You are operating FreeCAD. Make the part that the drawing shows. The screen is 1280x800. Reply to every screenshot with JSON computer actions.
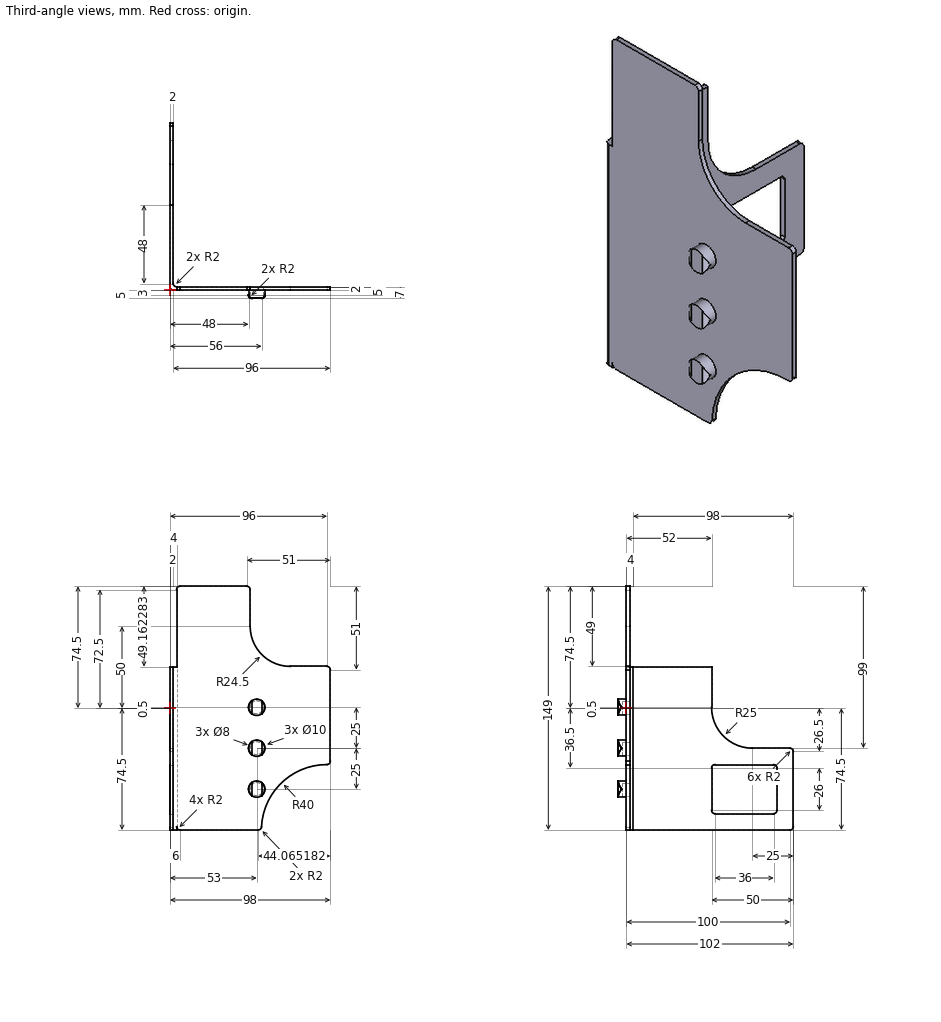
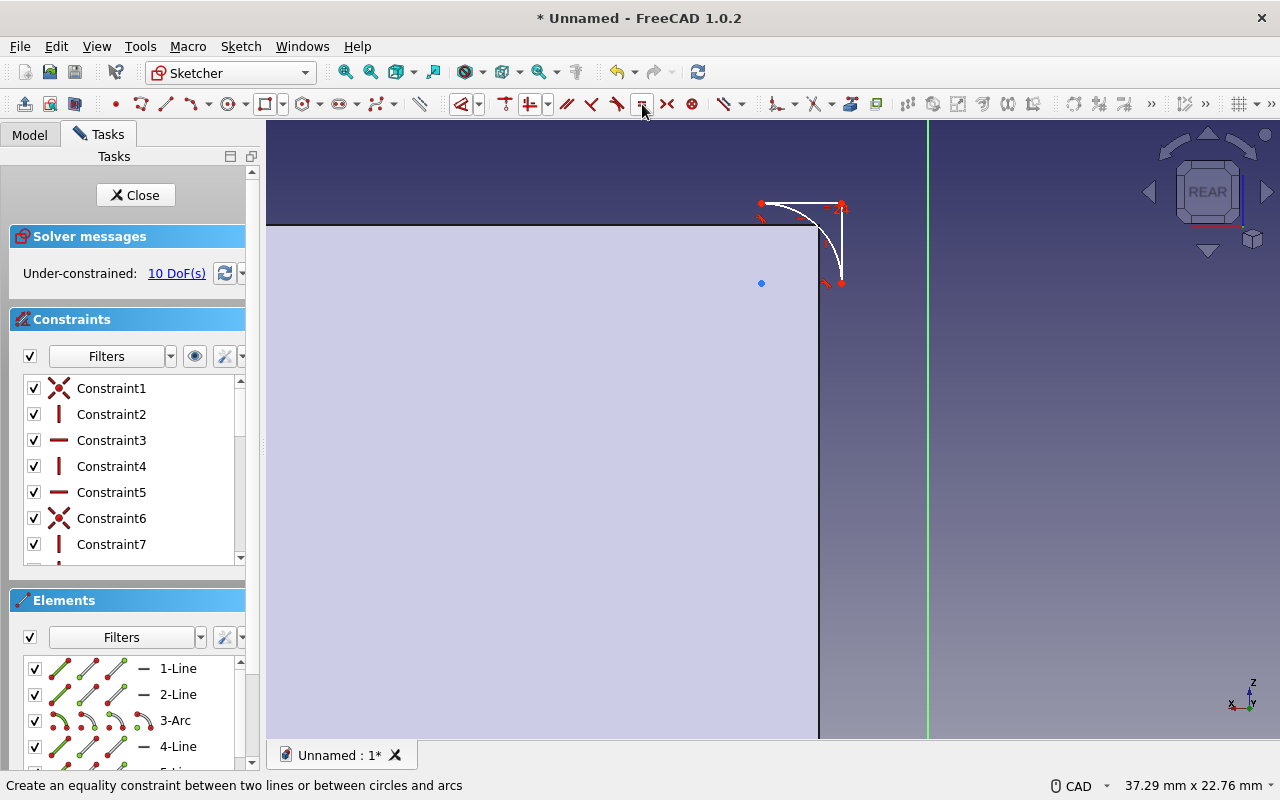
{"action": "scroll", "coordinate": [815, 248], "scroll_direction": "down", "scroll_amount": 12}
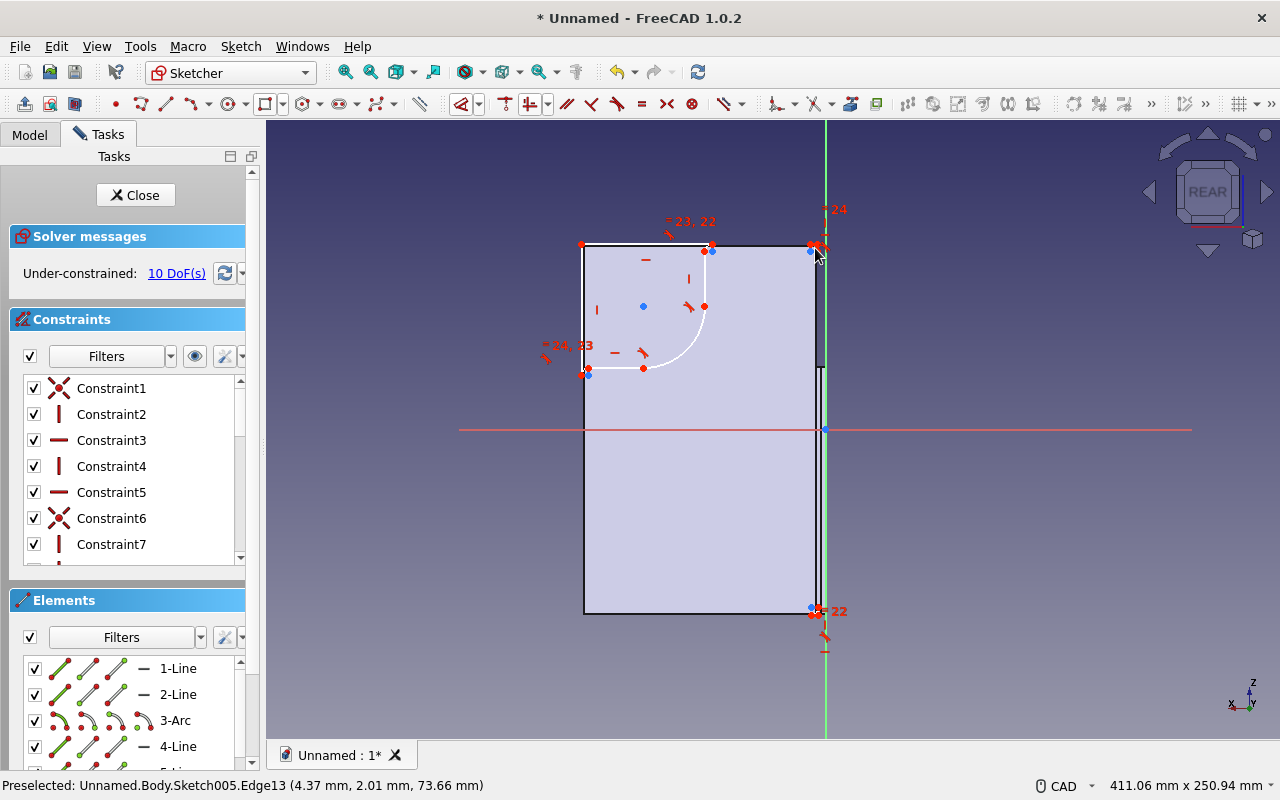
{"action": "scroll", "coordinate": [816, 613], "scroll_direction": "up", "scroll_amount": 11}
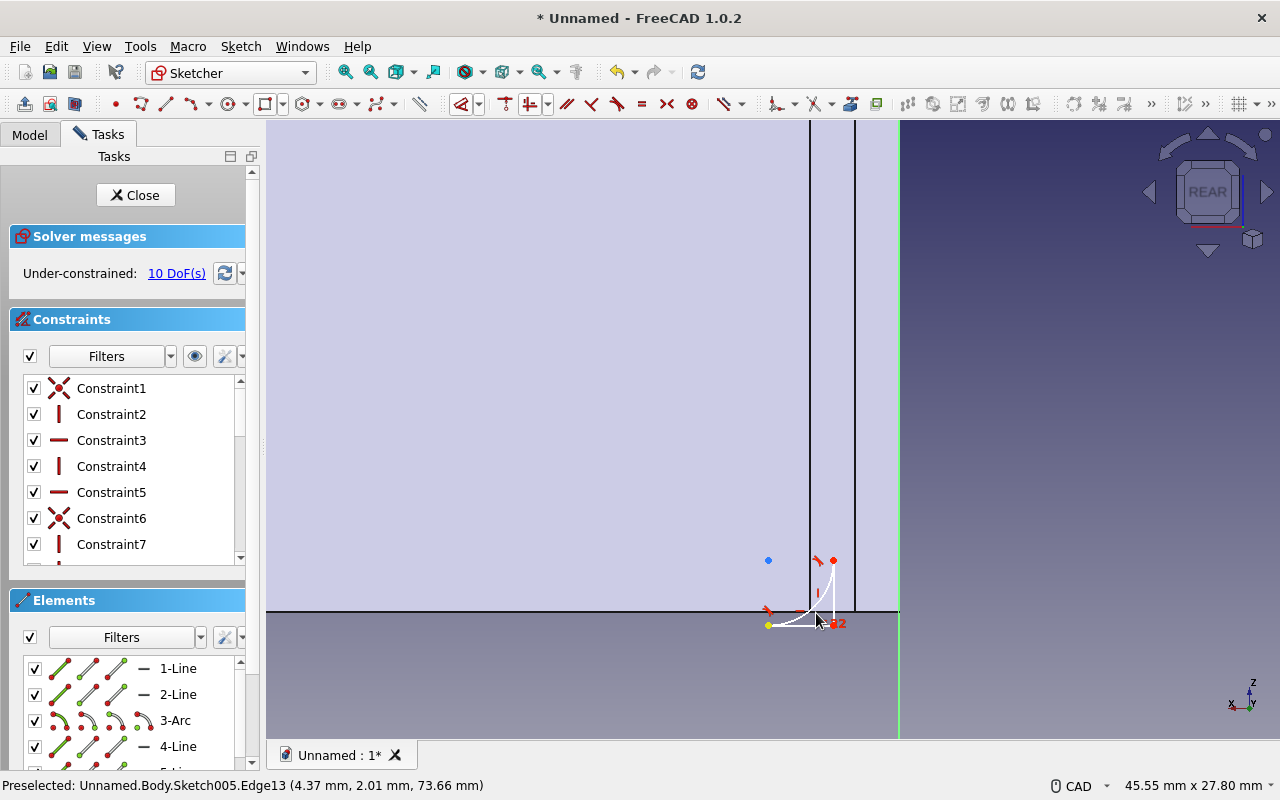
{"action": "left_click", "coordinate": [815, 606]}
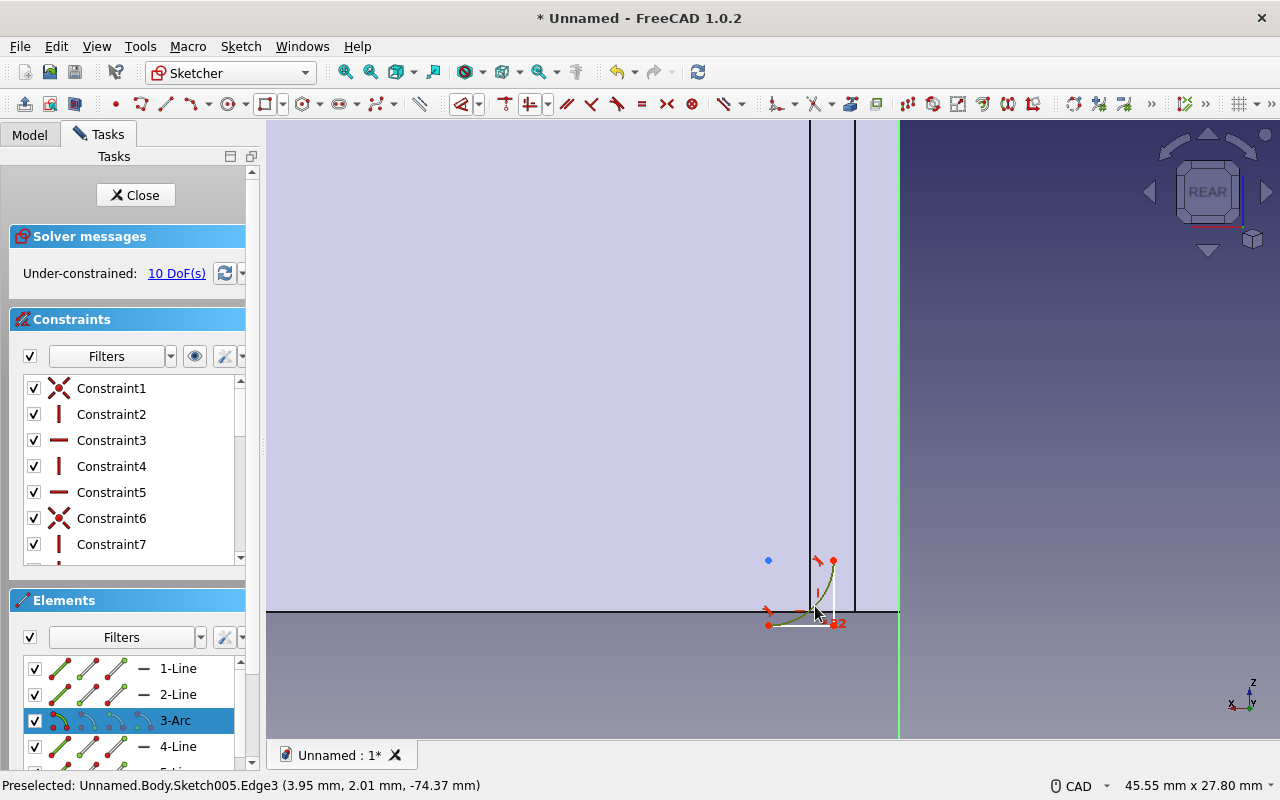
{"action": "key", "text": "k r"}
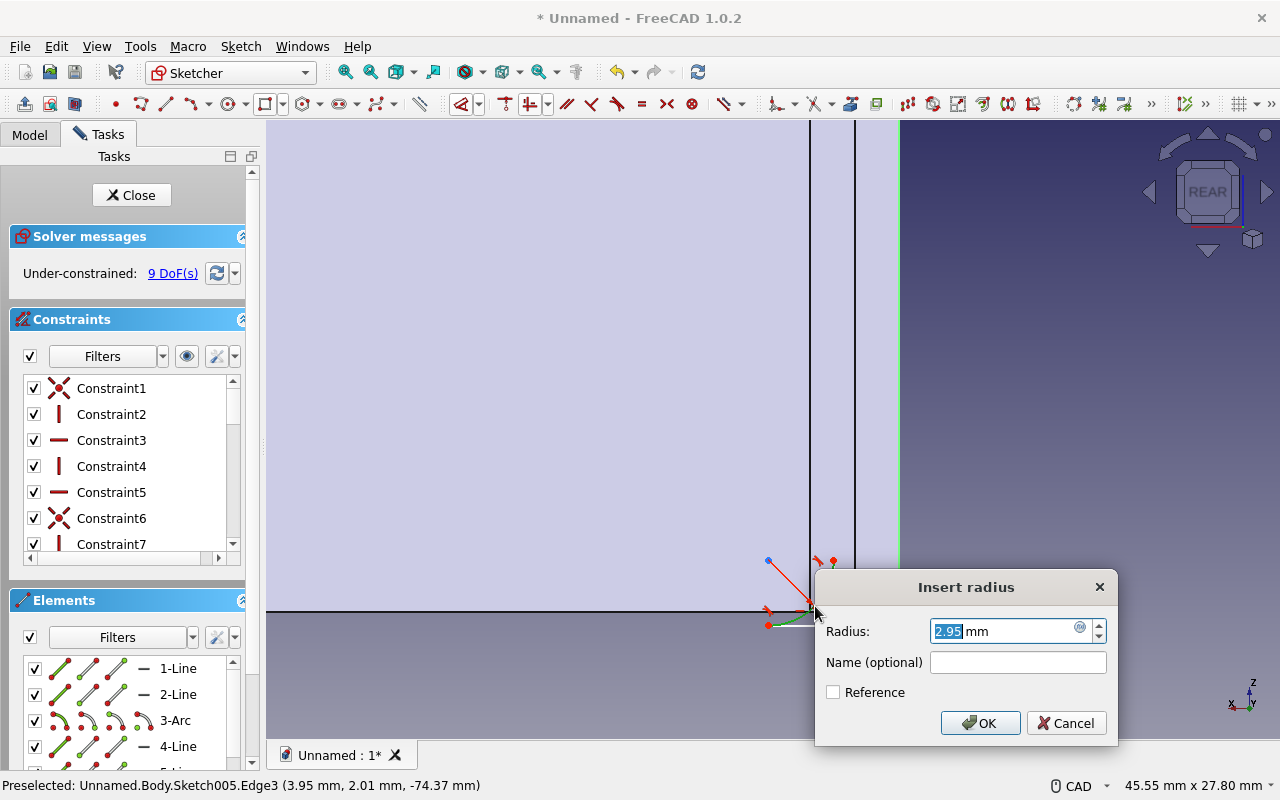
{"action": "type", "text": "2"}
{"action": "key", "text": "Return"}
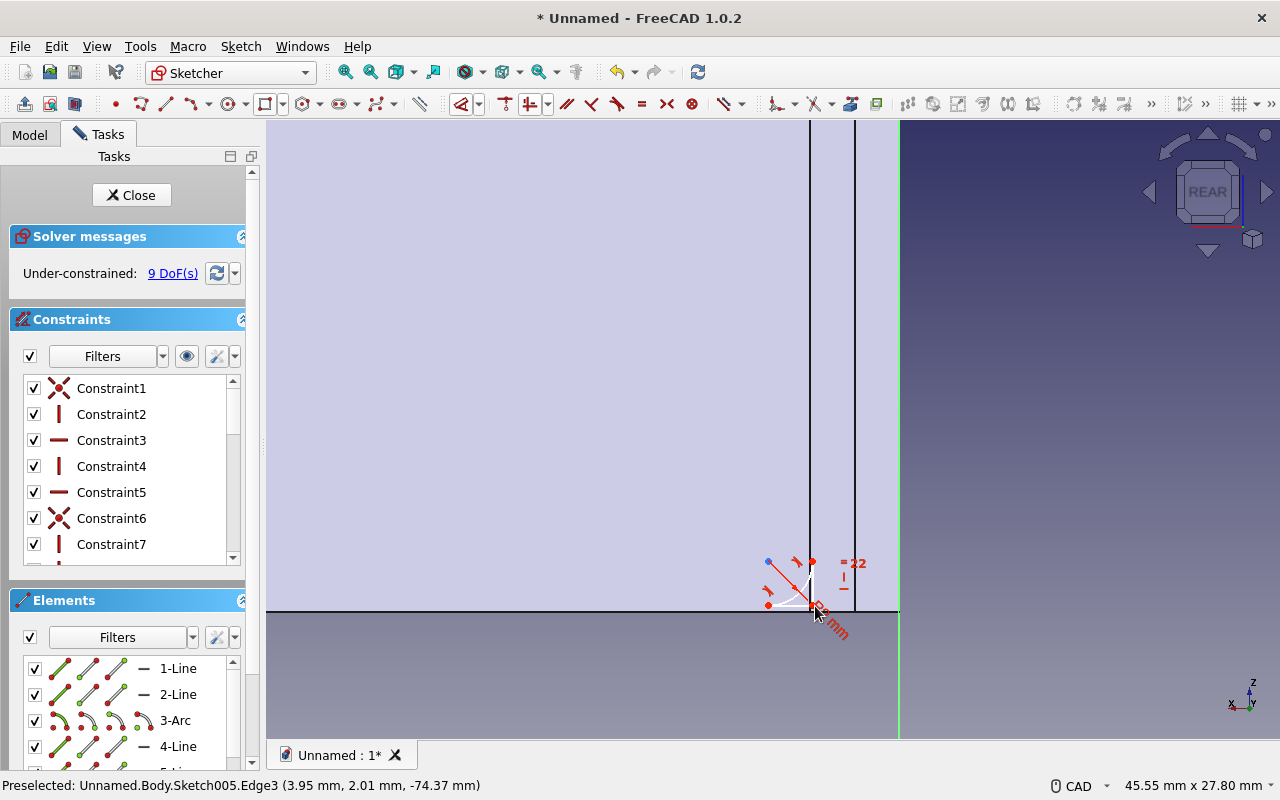
{"action": "scroll", "coordinate": [816, 613], "scroll_direction": "down", "scroll_amount": 11}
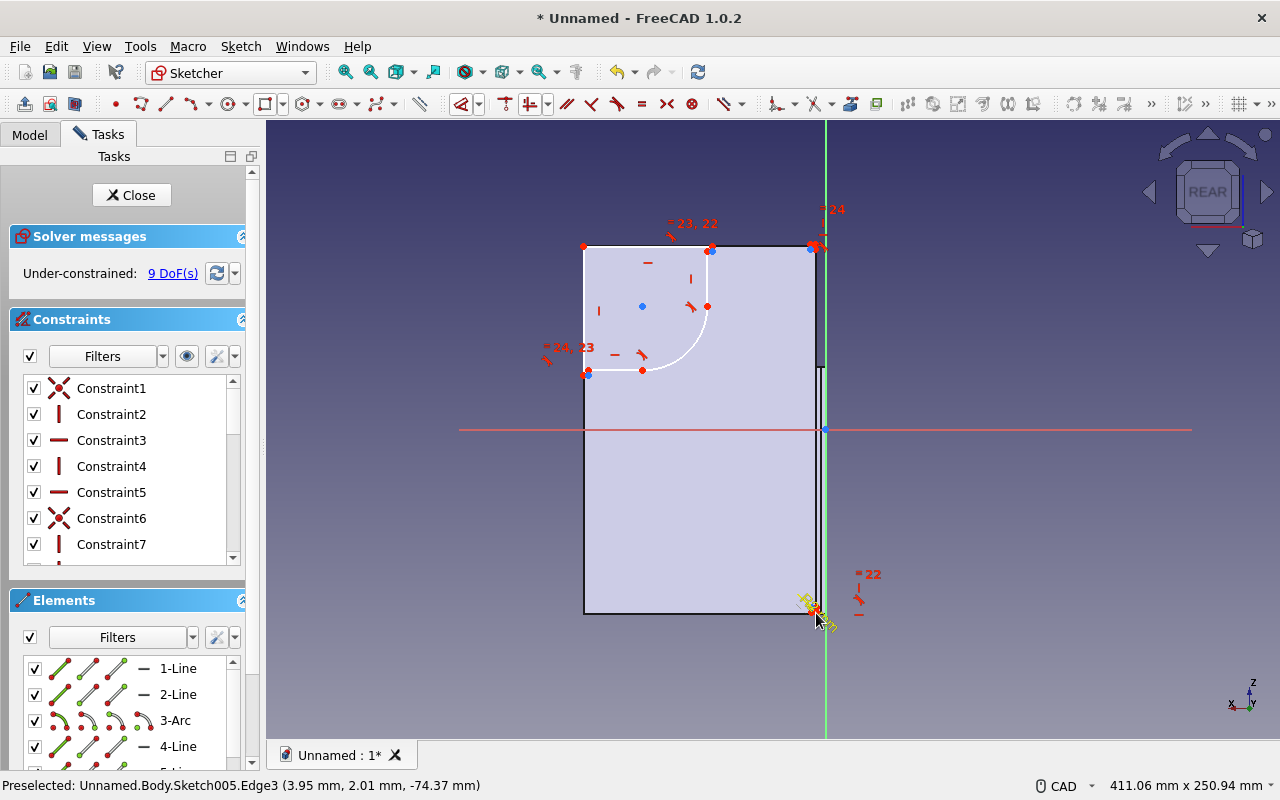
{"action": "left_click", "coordinate": [672, 363]}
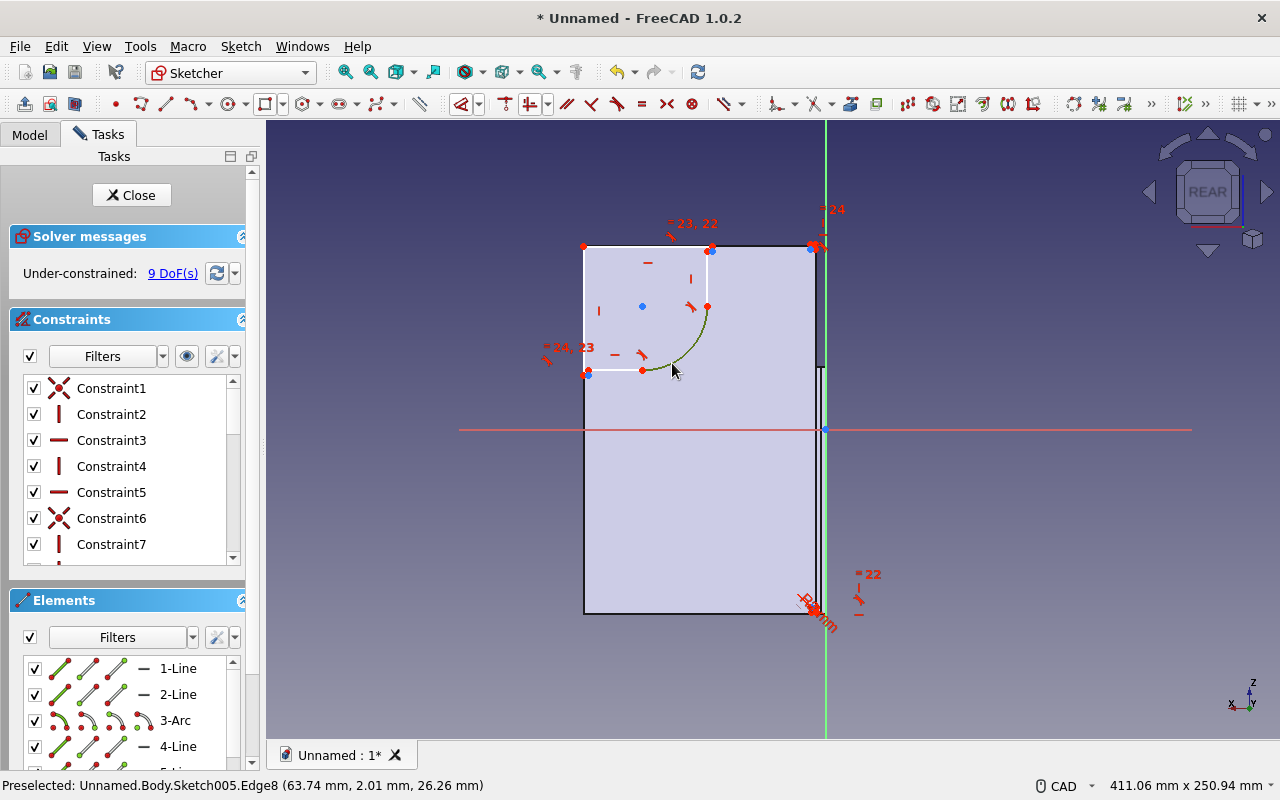
{"action": "key", "text": "k r"}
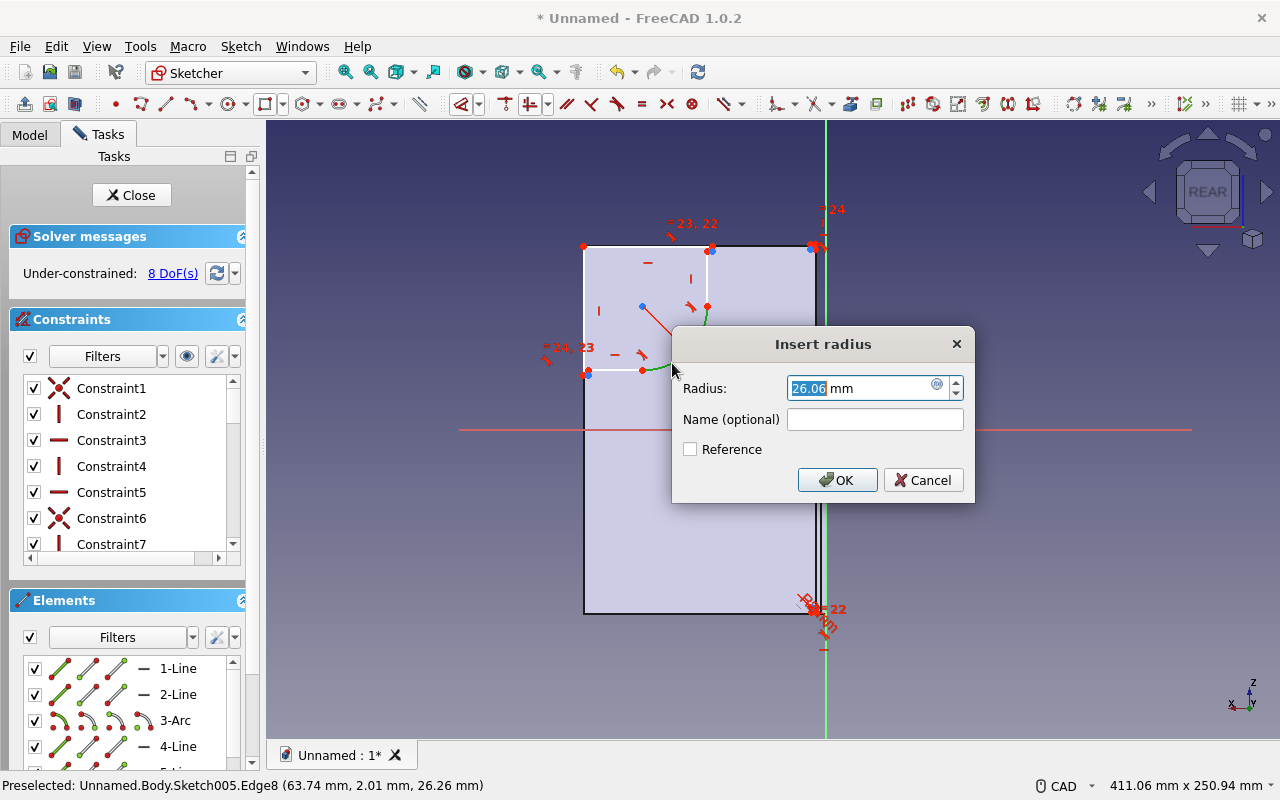
{"action": "type", "text": "24.5"}
{"action": "key", "text": "Return"}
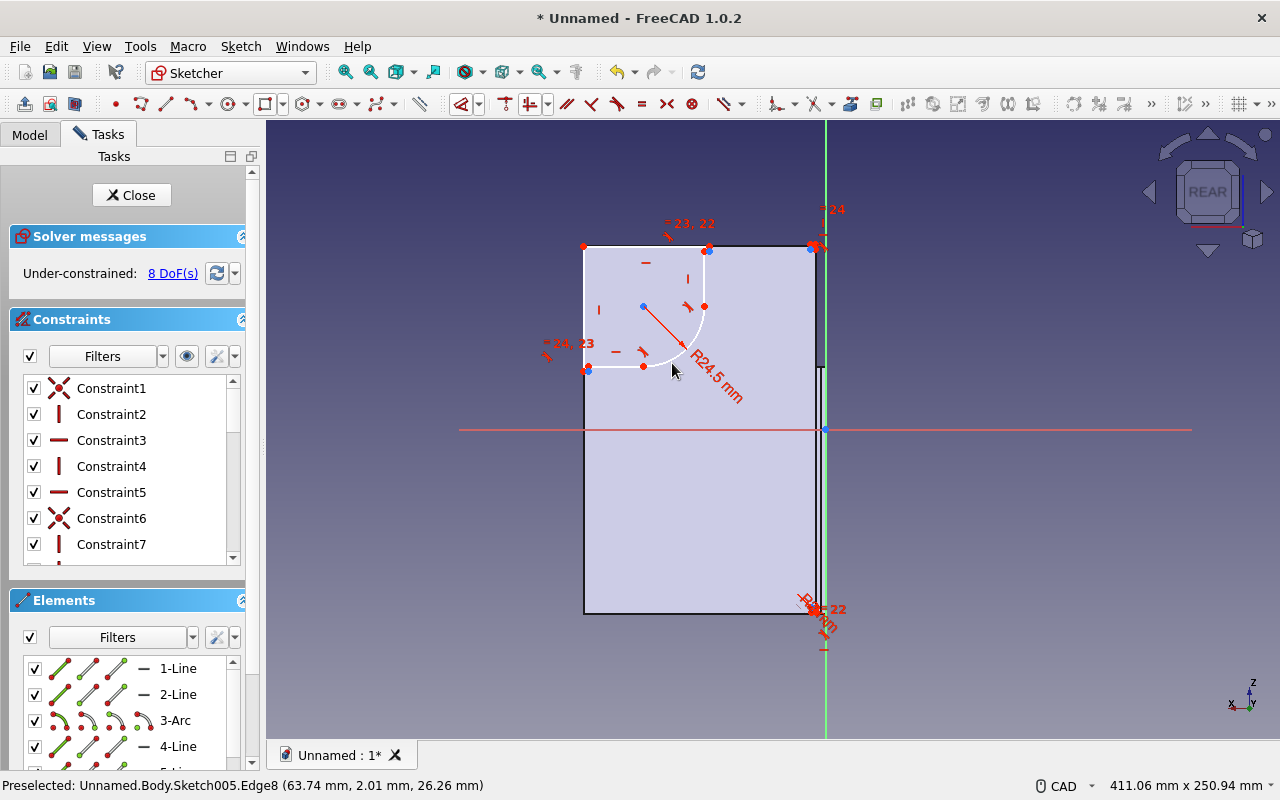
{"action": "left_click", "coordinate": [672, 247]}